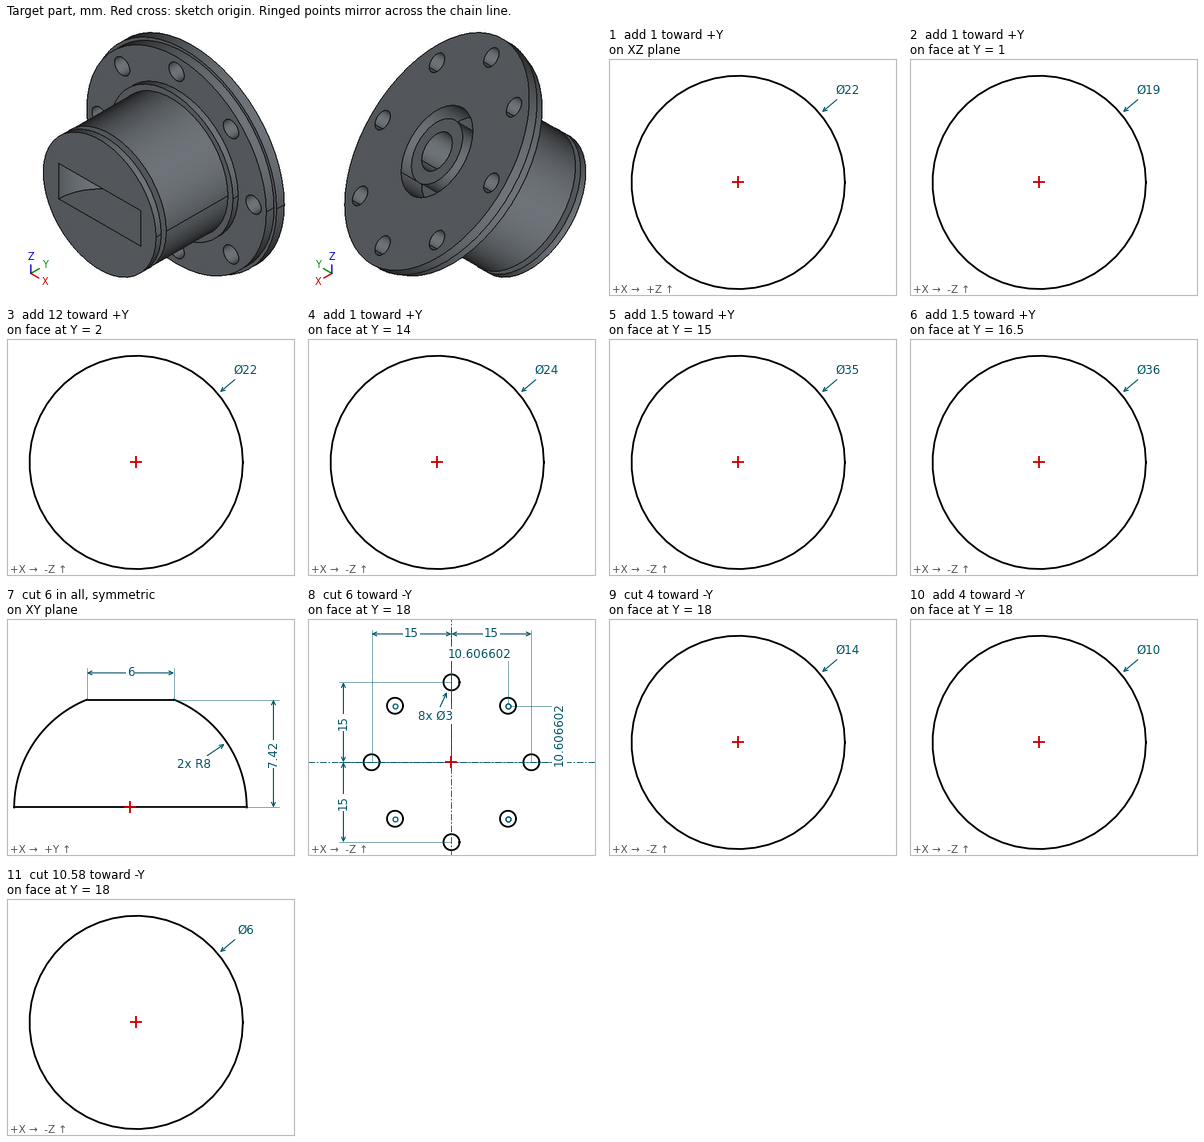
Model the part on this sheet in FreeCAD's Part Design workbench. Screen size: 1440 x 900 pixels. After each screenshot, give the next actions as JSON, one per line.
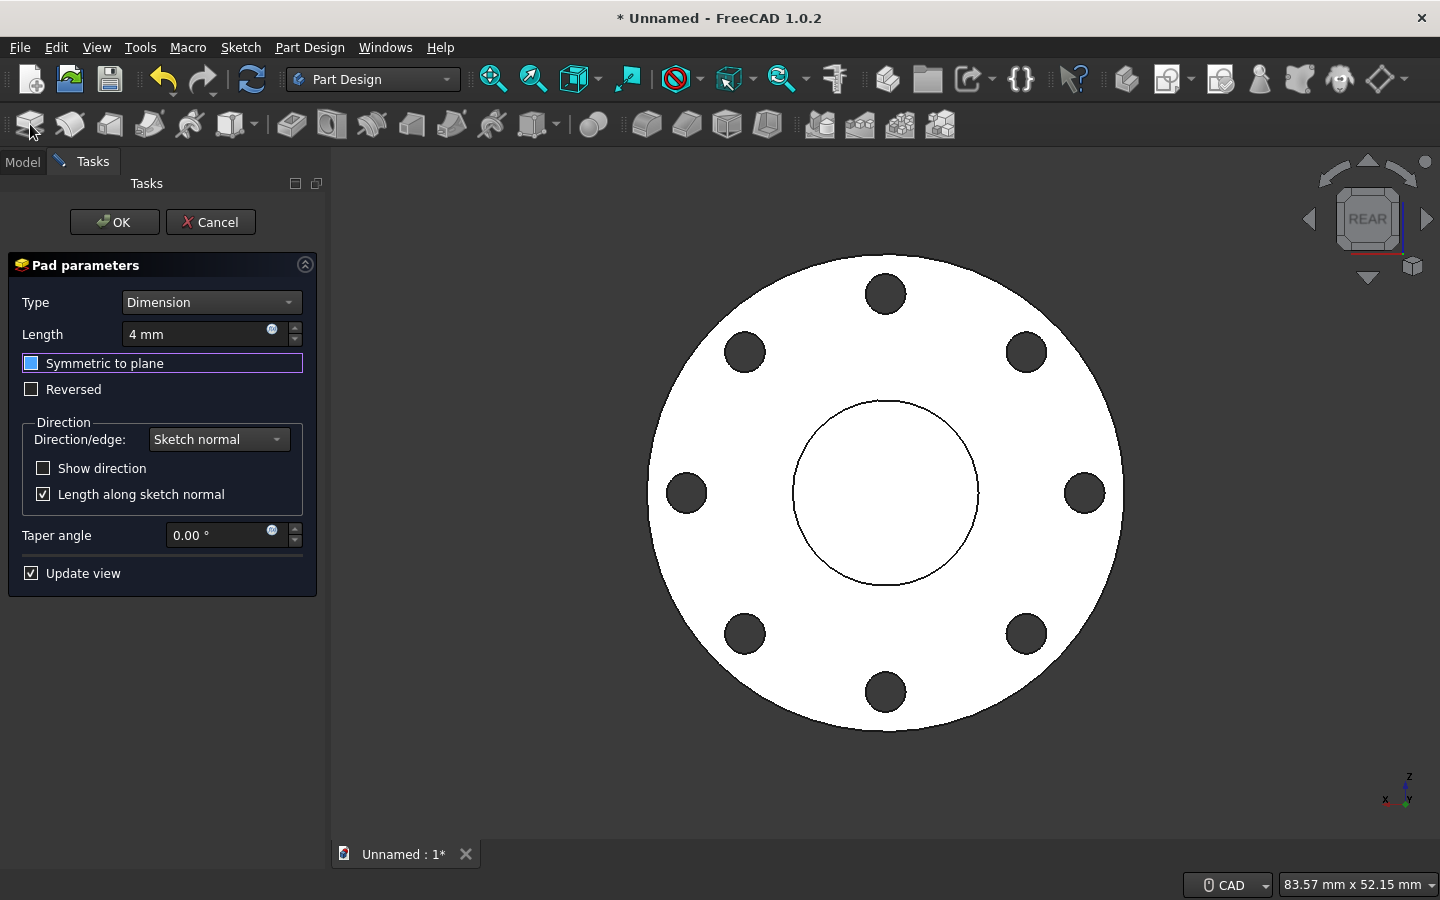
{"action": "left_click", "coordinate": [30, 389]}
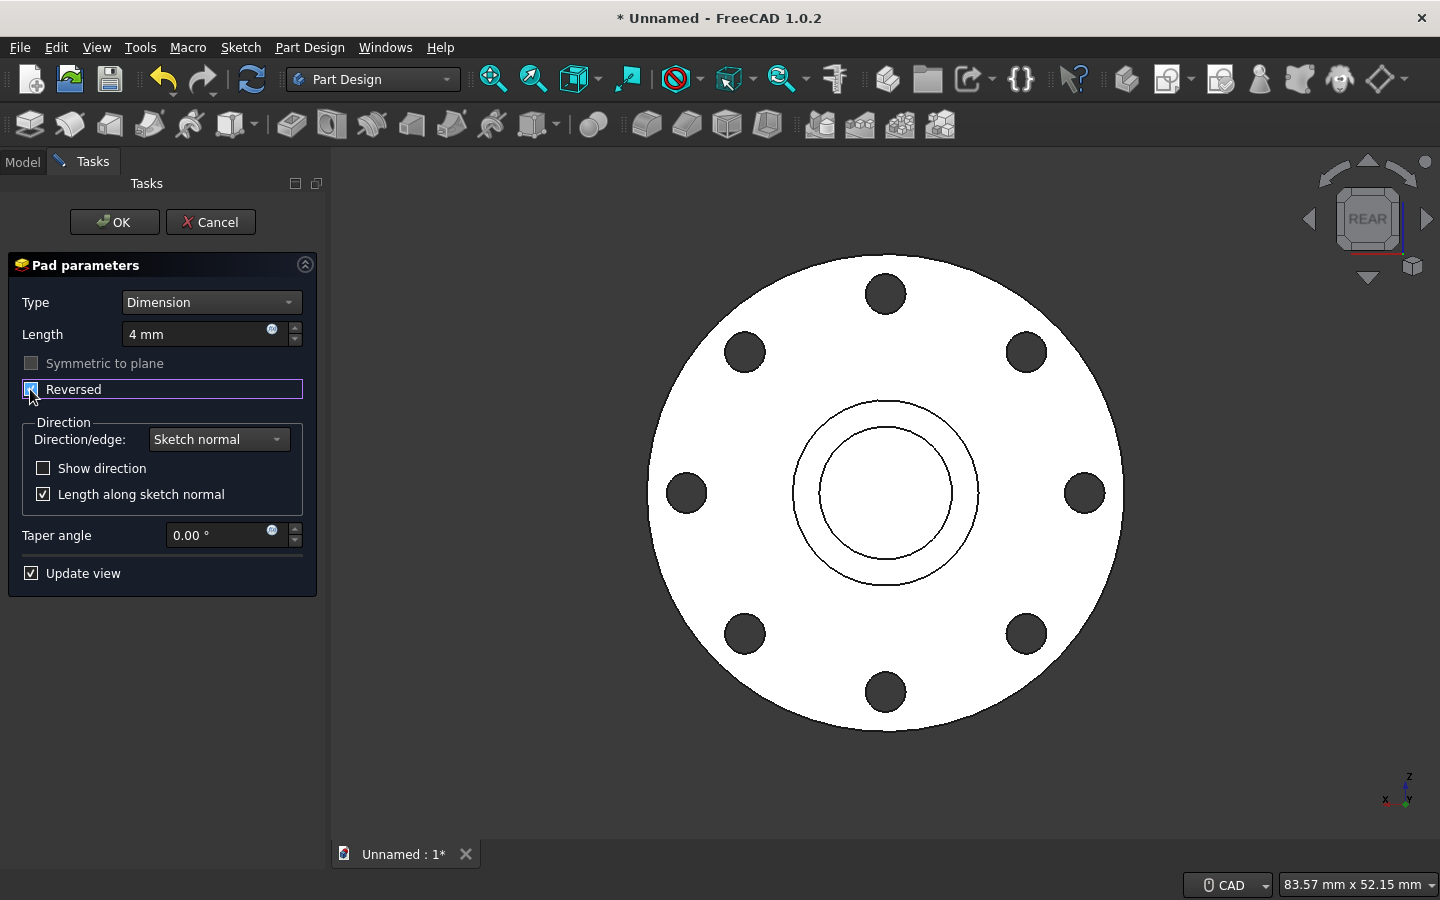
{"action": "left_click", "coordinate": [115, 222]}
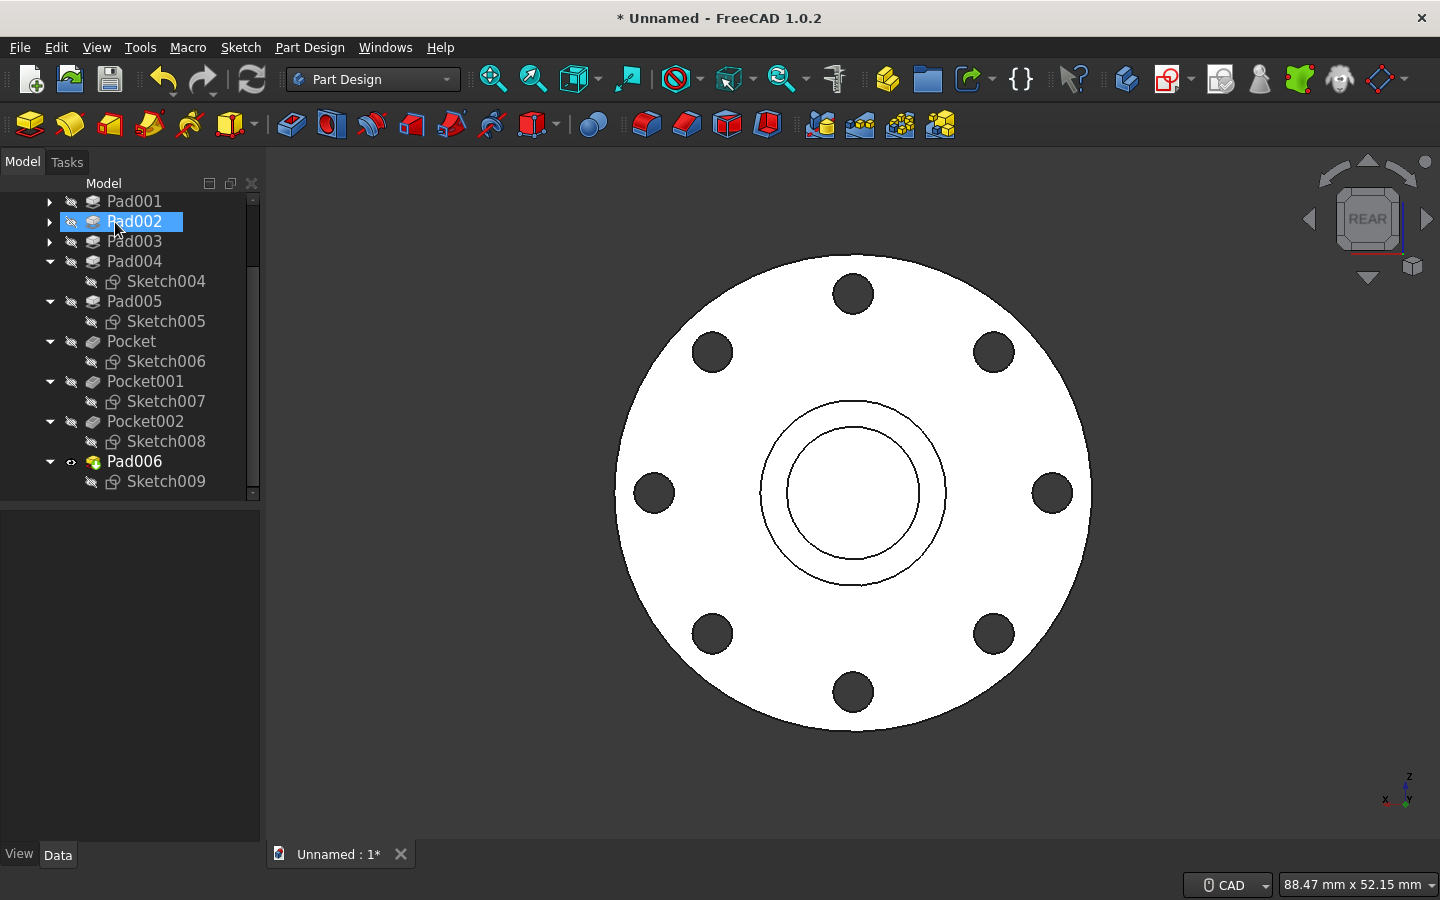
{"action": "left_click", "coordinate": [785, 628]}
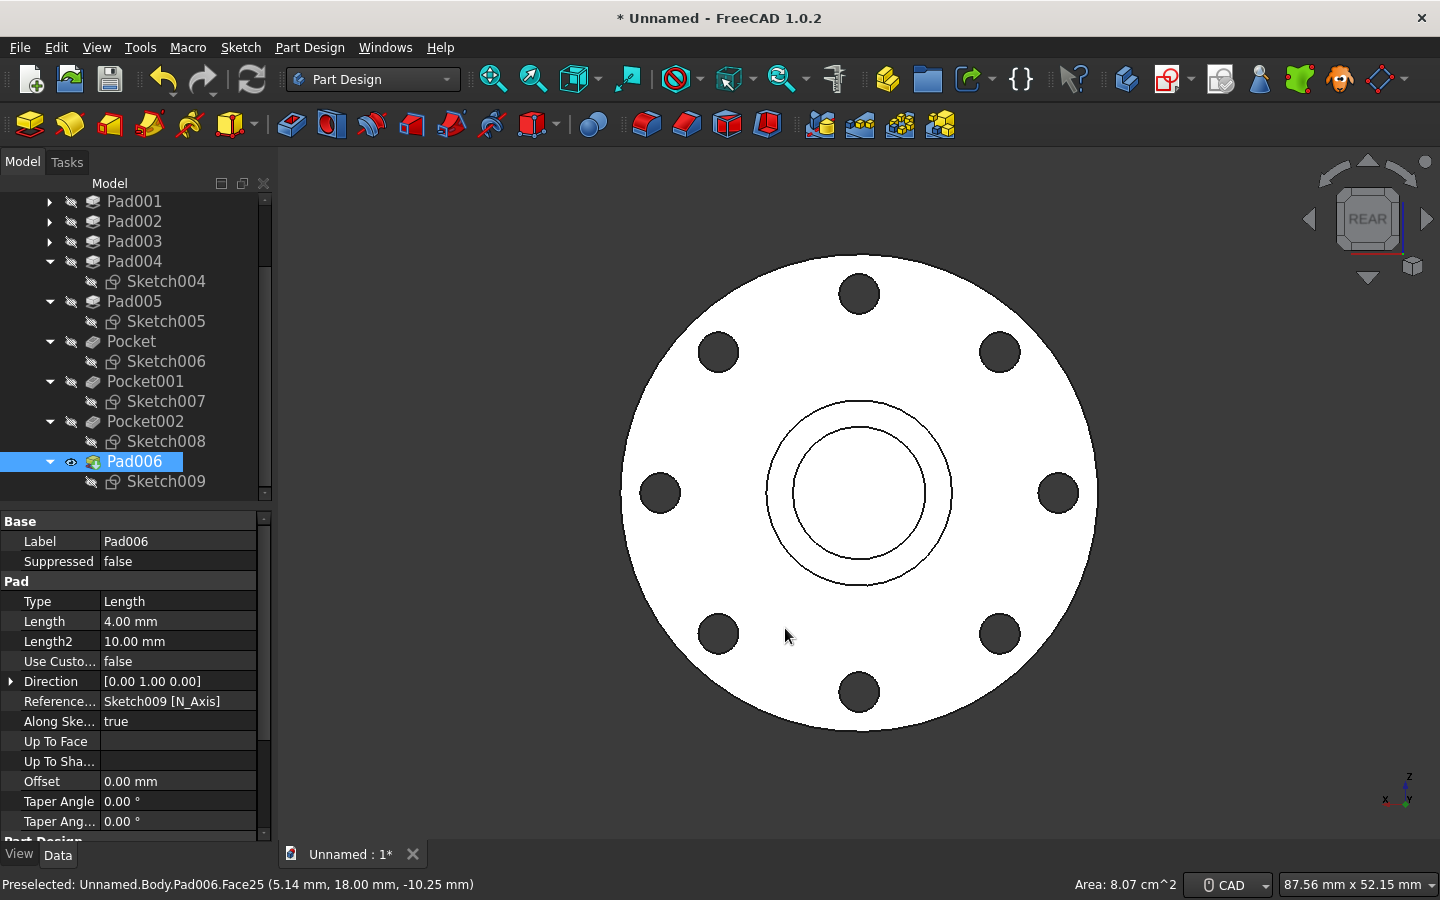
{"action": "left_click", "coordinate": [1168, 80]}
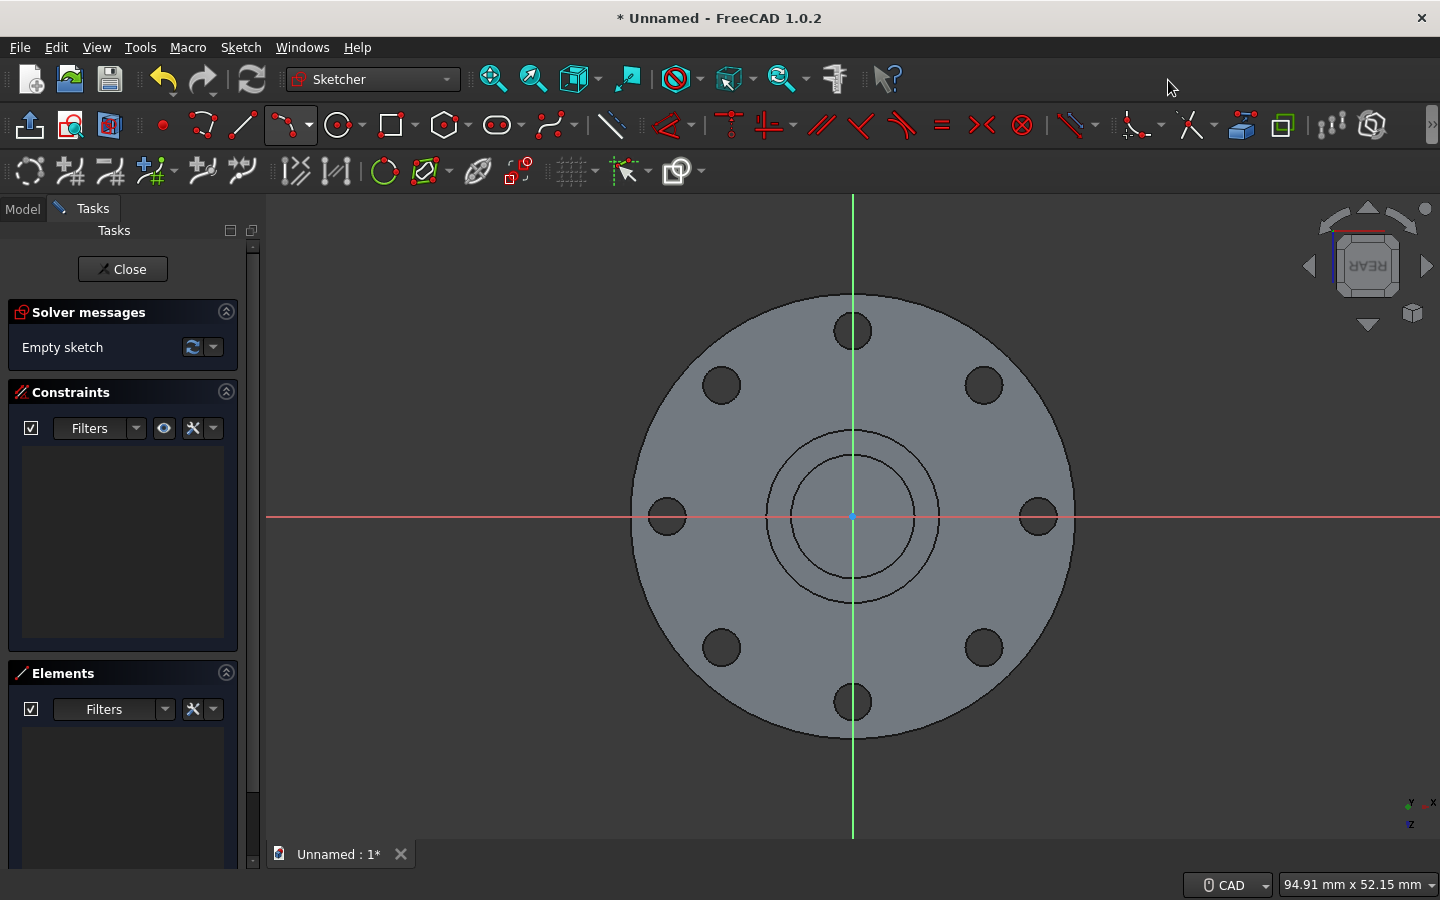
{"action": "scroll", "coordinate": [866, 516], "scroll_direction": "up", "scroll_amount": 9}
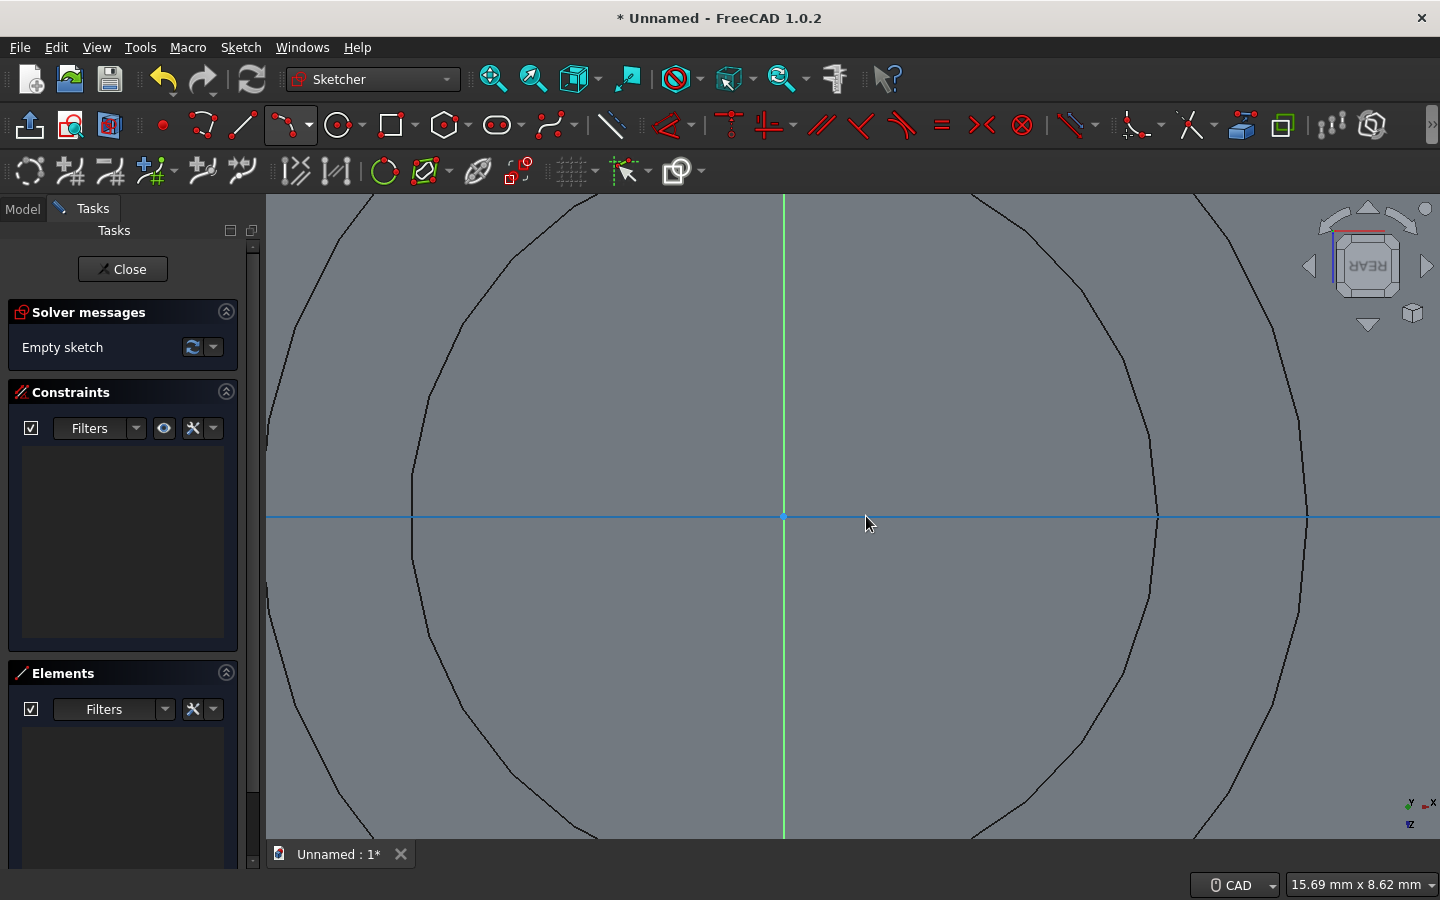
{"action": "left_click", "coordinate": [338, 126]}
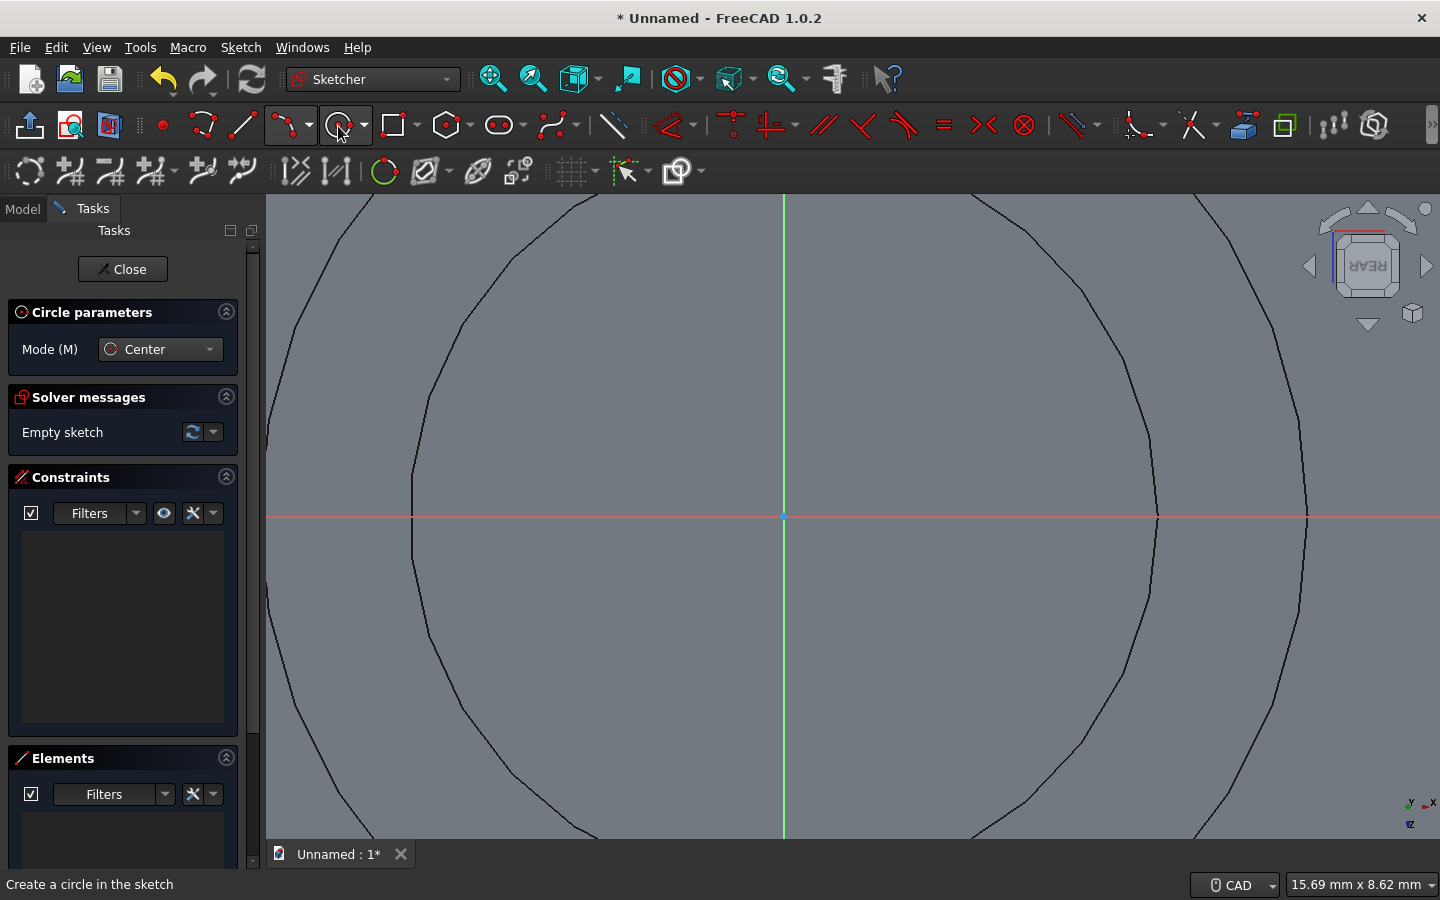
{"action": "left_click", "coordinate": [784, 516]}
{"action": "mouse_move", "coordinate": [942, 358]}